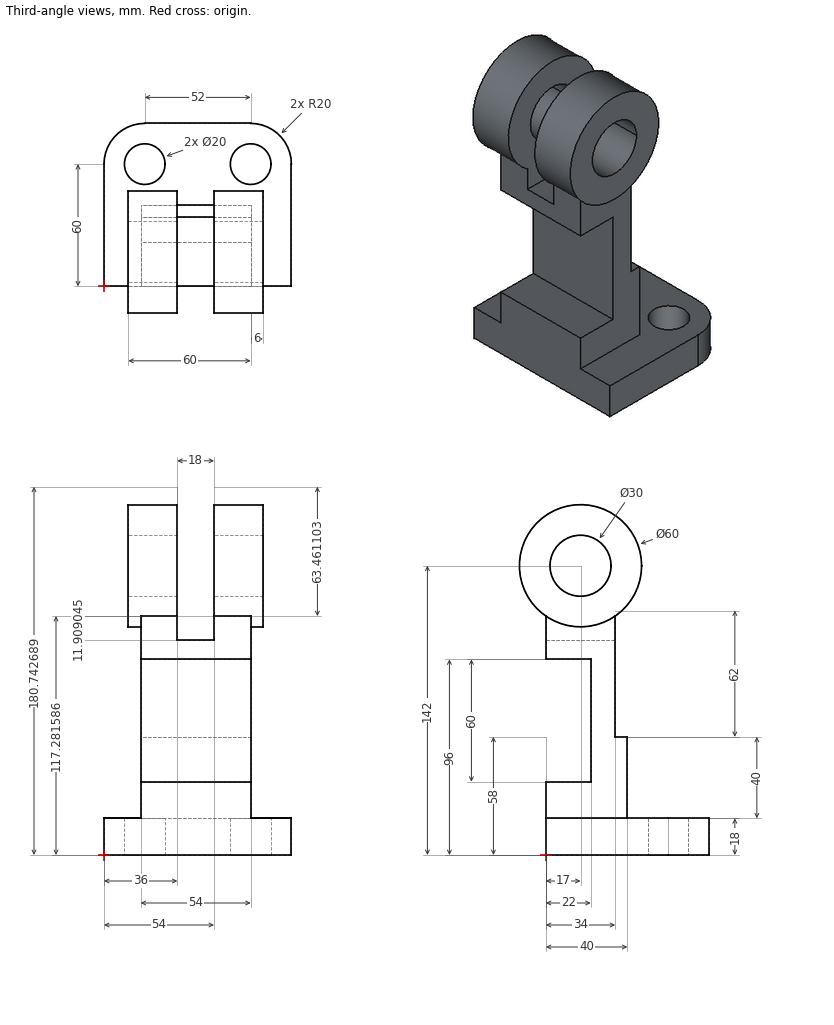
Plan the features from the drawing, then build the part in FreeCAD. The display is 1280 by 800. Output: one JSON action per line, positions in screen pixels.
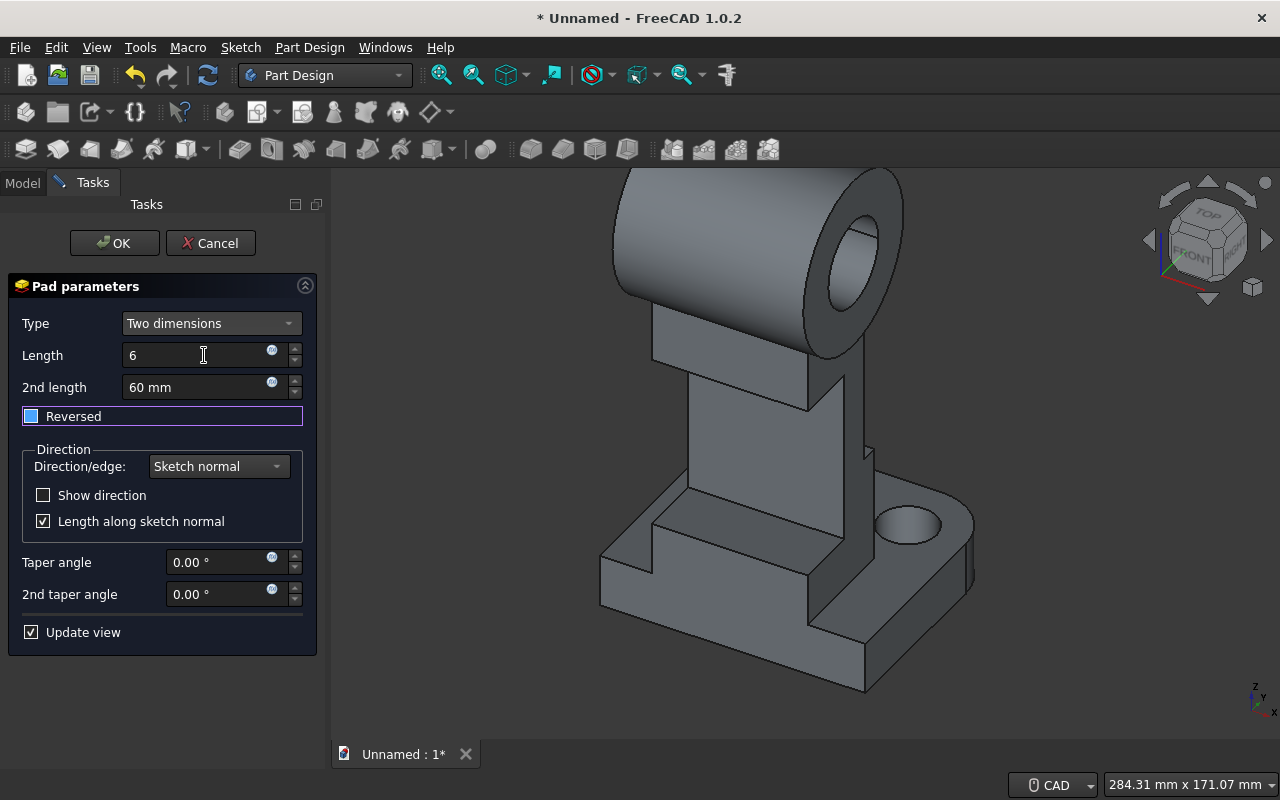
{"action": "left_click", "coordinate": [115, 243]}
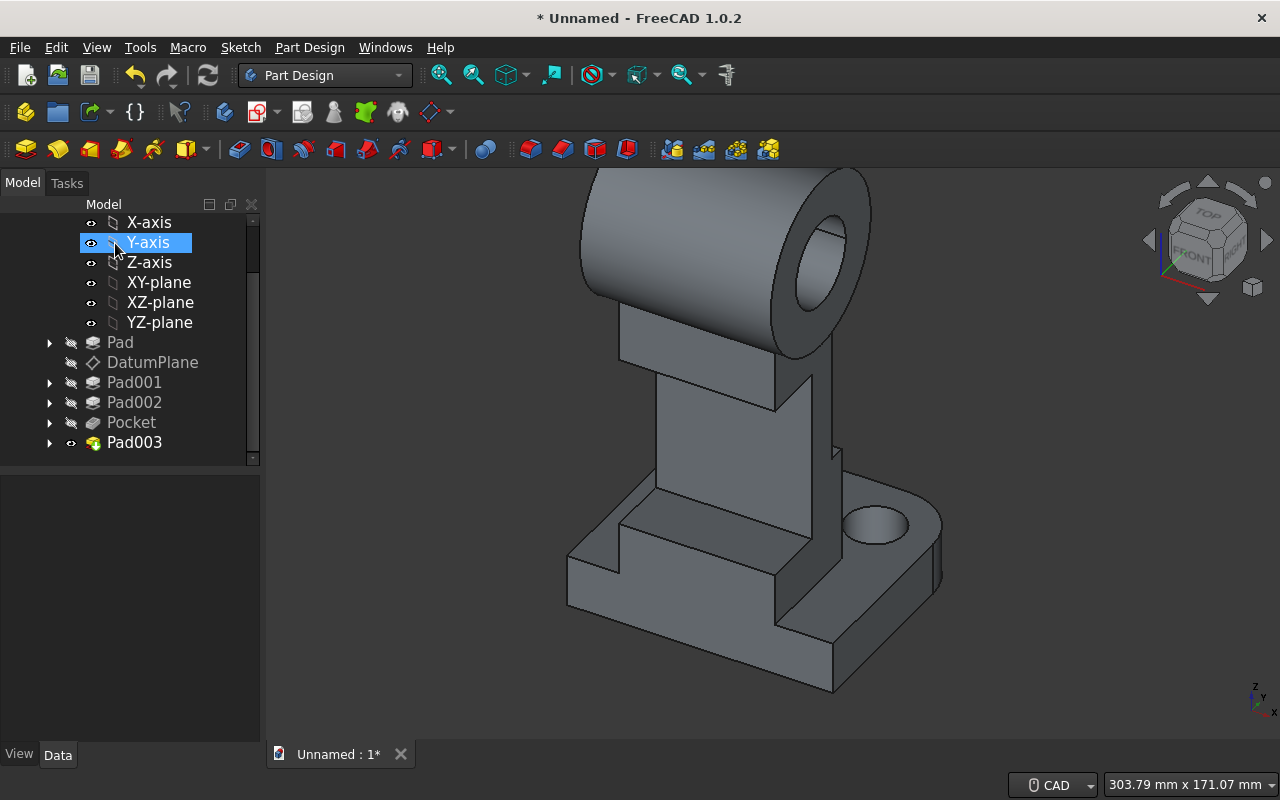
{"action": "left_click", "coordinate": [442, 76]}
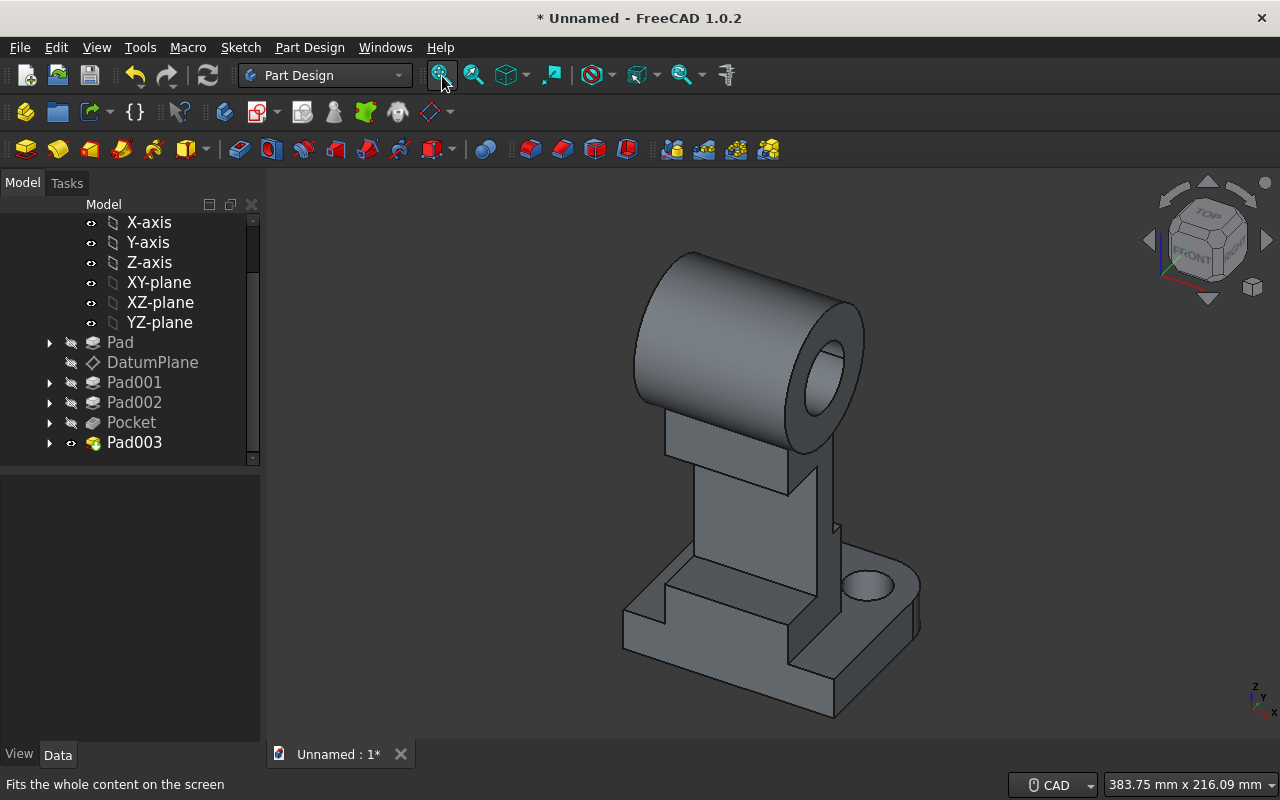
{"action": "left_click", "coordinate": [258, 112]}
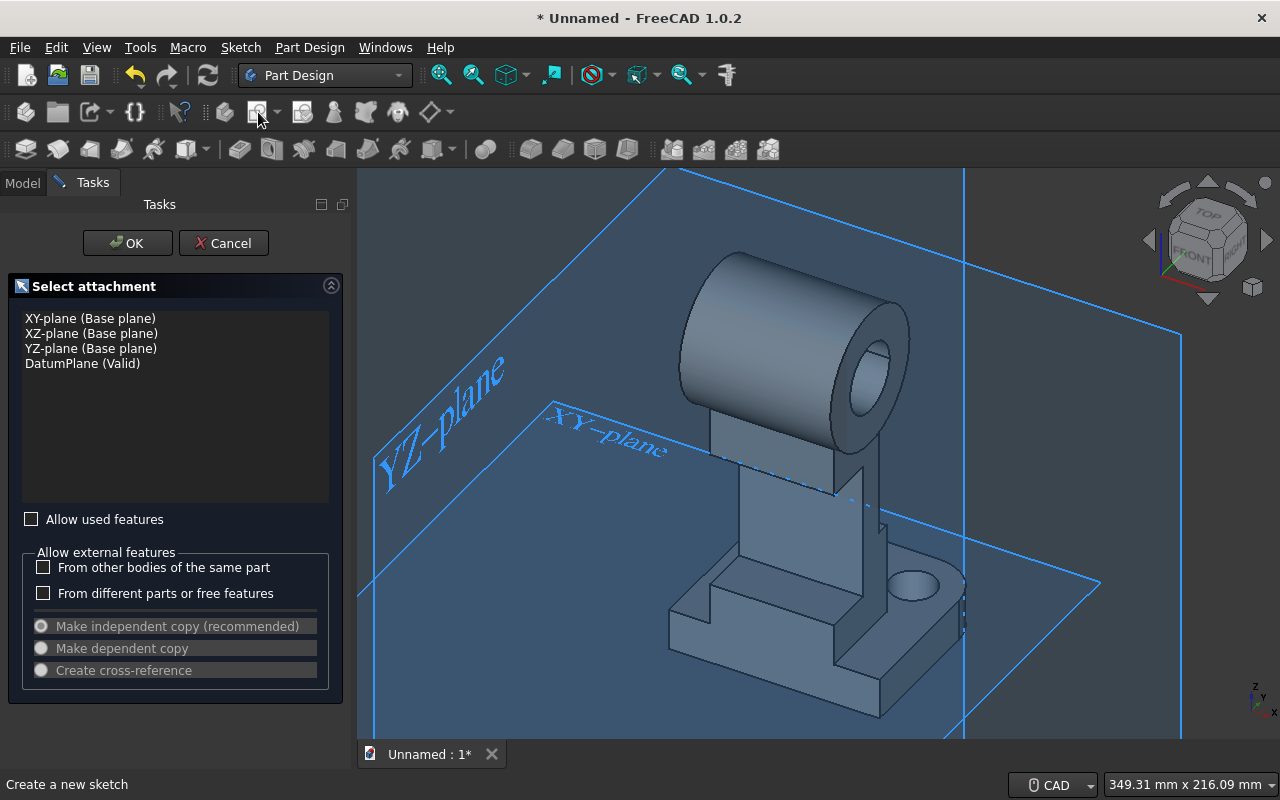
{"action": "left_click", "coordinate": [82, 334]}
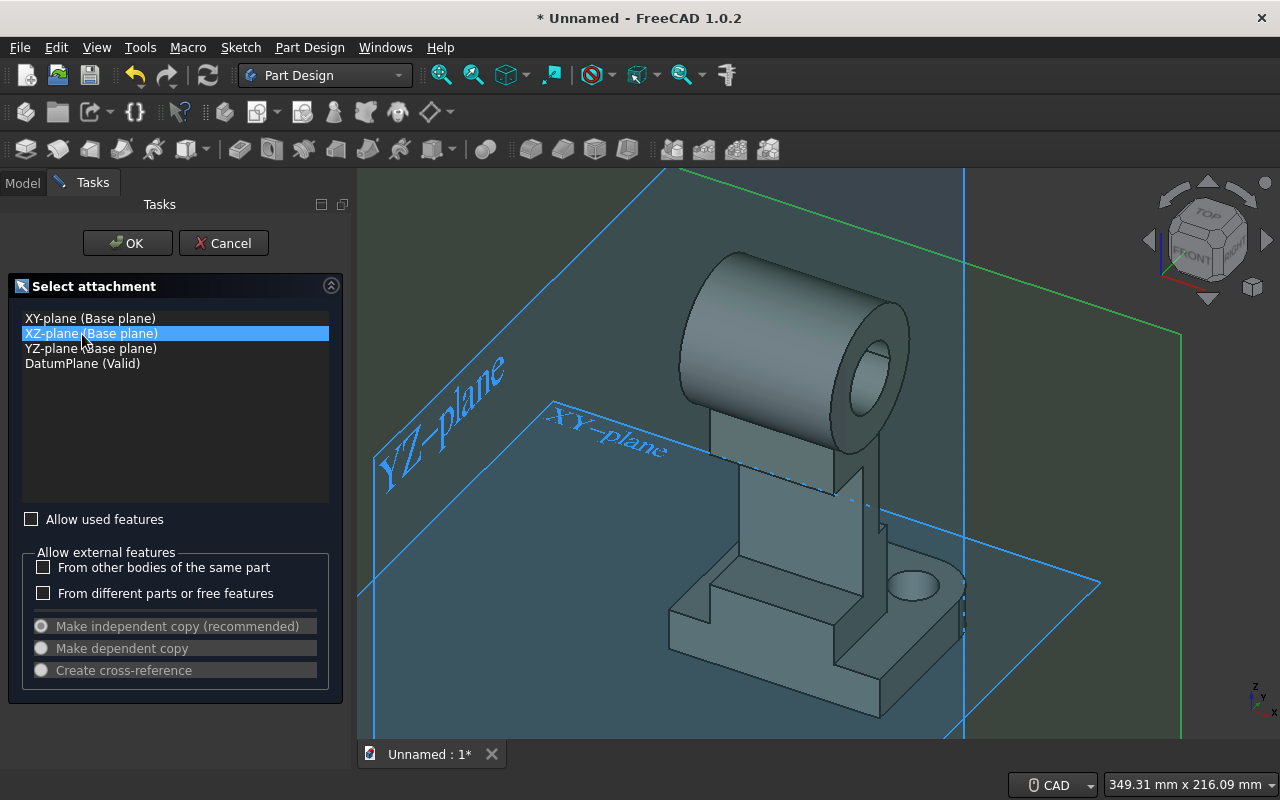
{"action": "left_click", "coordinate": [128, 243]}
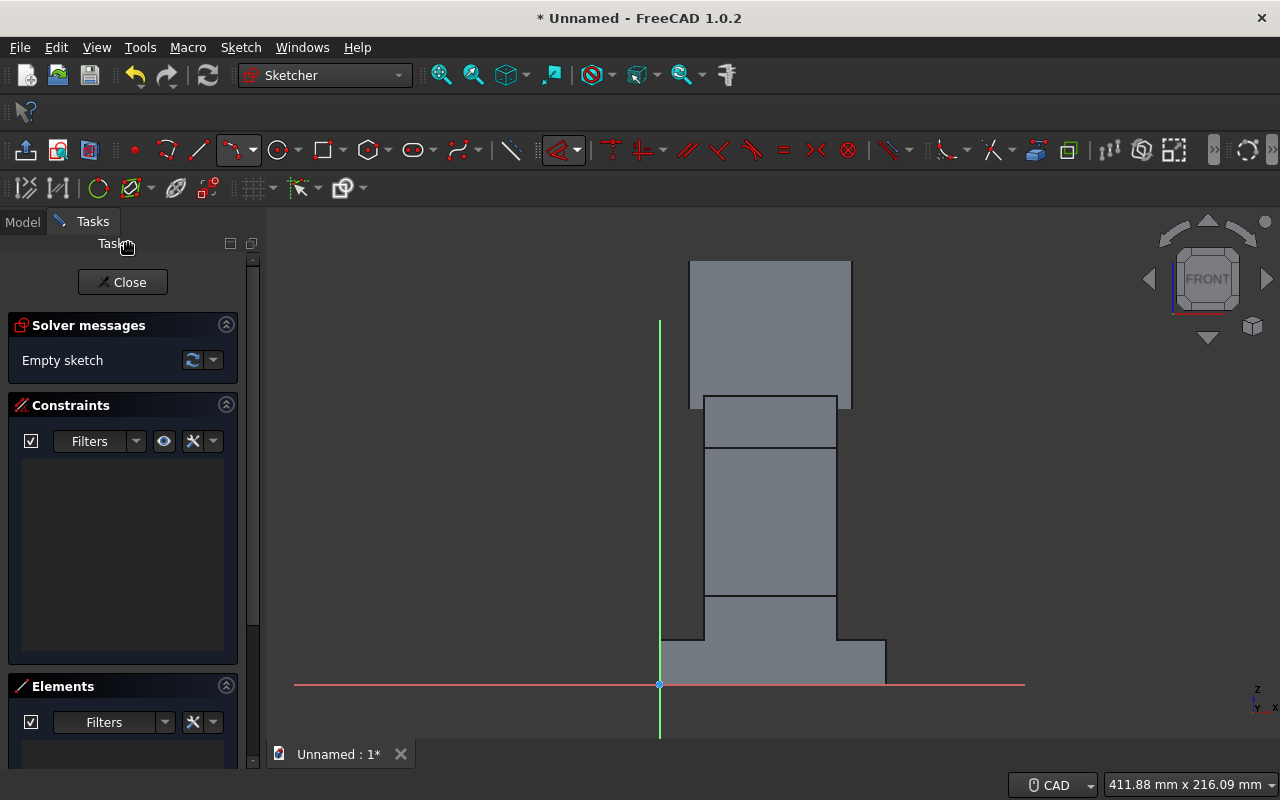
{"action": "left_click", "coordinate": [90, 150]}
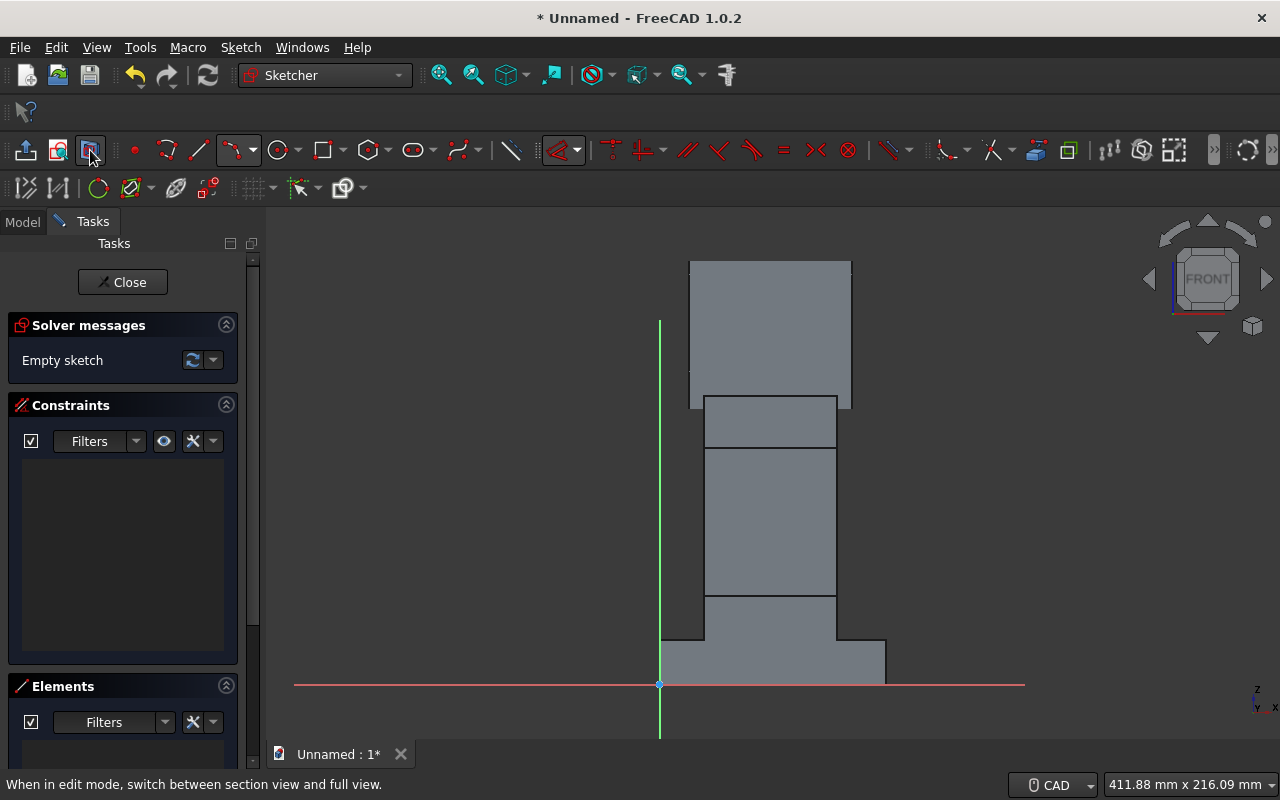
{"action": "scroll", "coordinate": [704, 473], "scroll_direction": "down", "scroll_amount": 5}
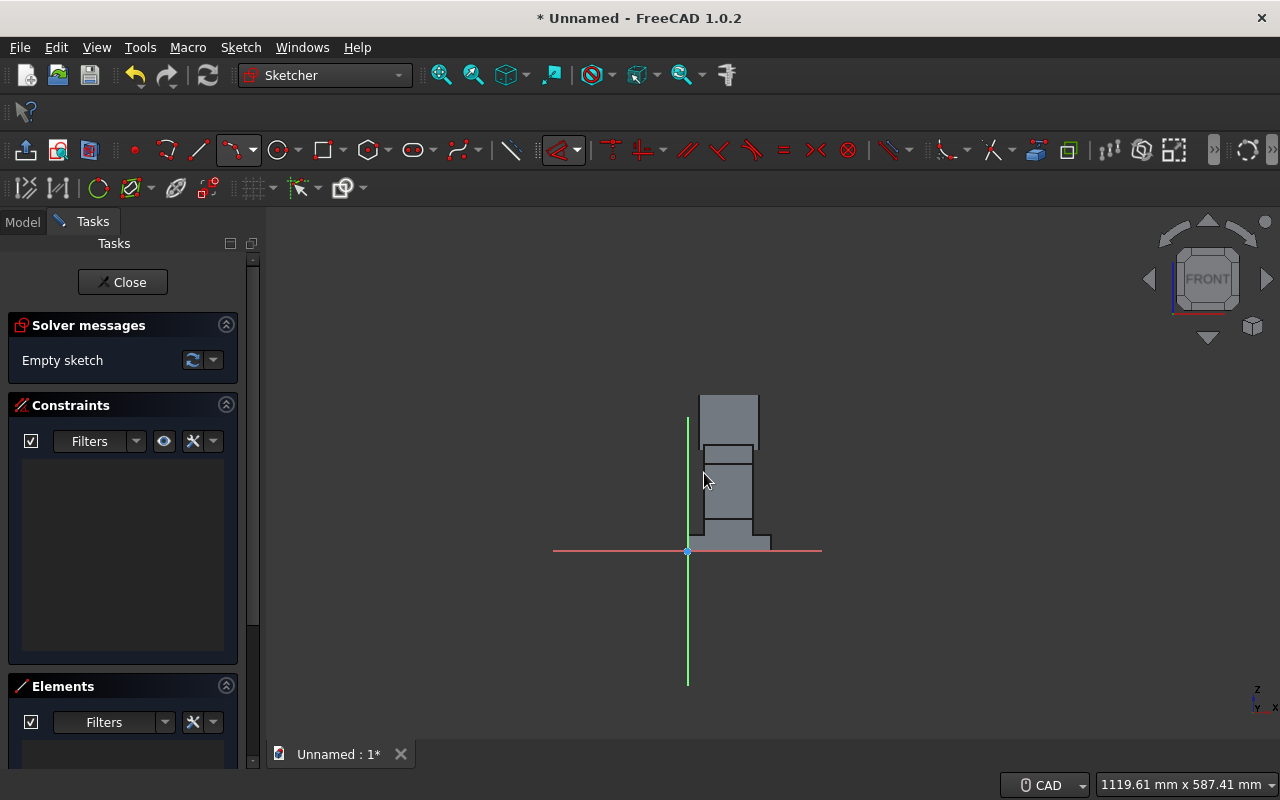
{"action": "scroll", "coordinate": [734, 405], "scroll_direction": "up", "scroll_amount": 9}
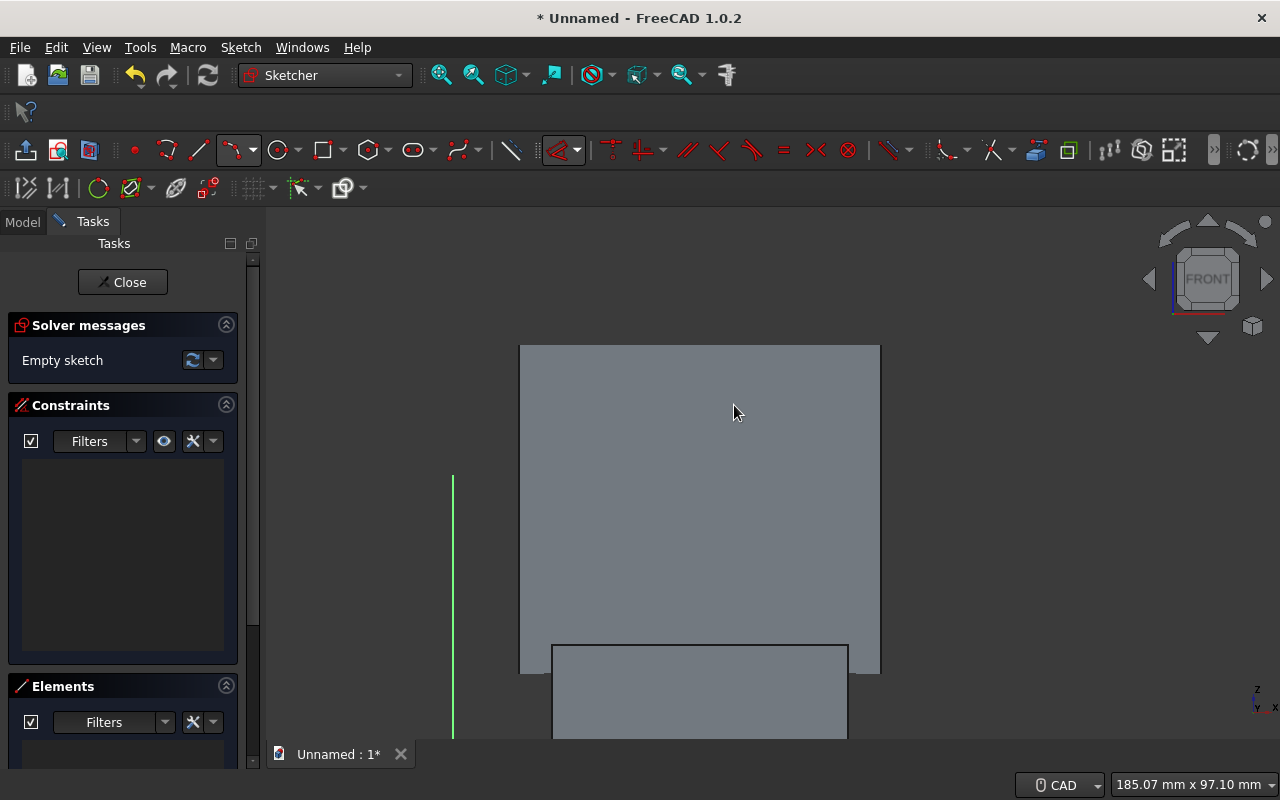
{"action": "left_click", "coordinate": [324, 150]}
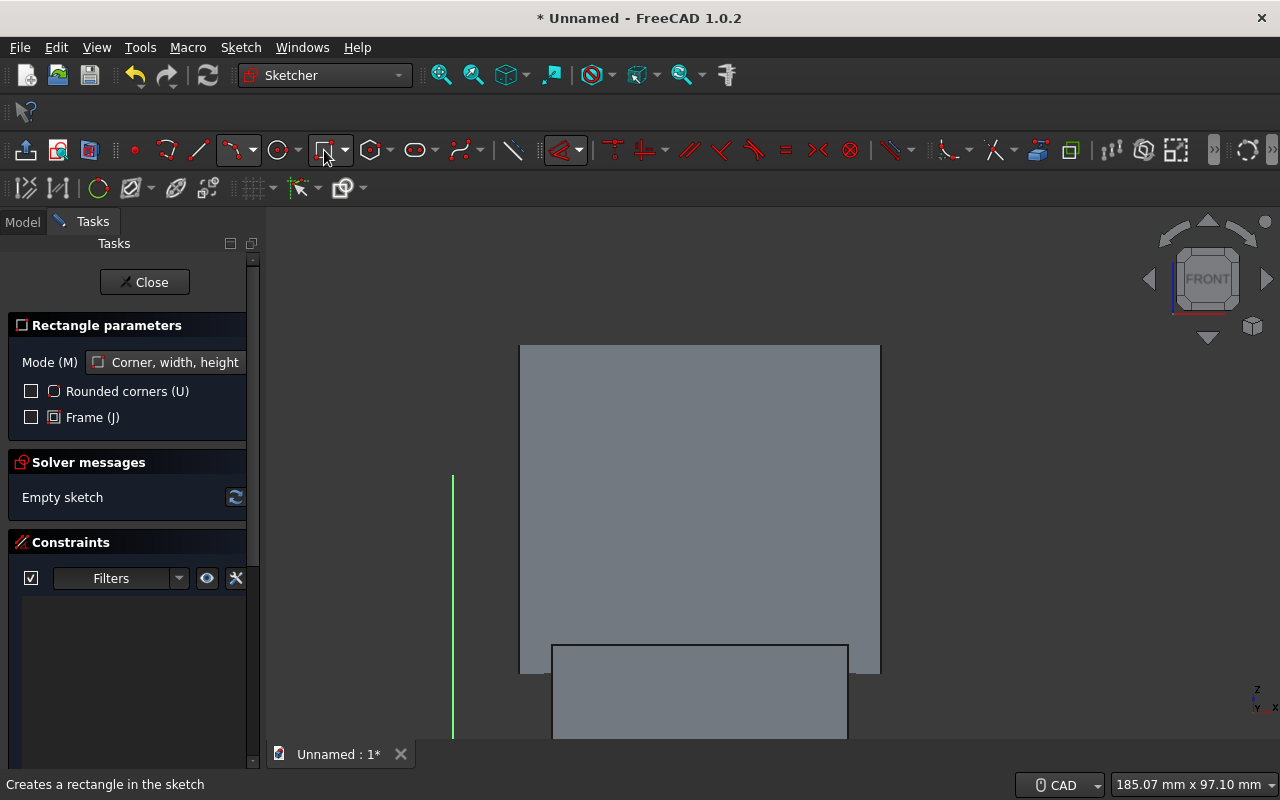
{"action": "left_click", "coordinate": [651, 297]}
{"action": "mouse_move", "coordinate": [749, 645]}